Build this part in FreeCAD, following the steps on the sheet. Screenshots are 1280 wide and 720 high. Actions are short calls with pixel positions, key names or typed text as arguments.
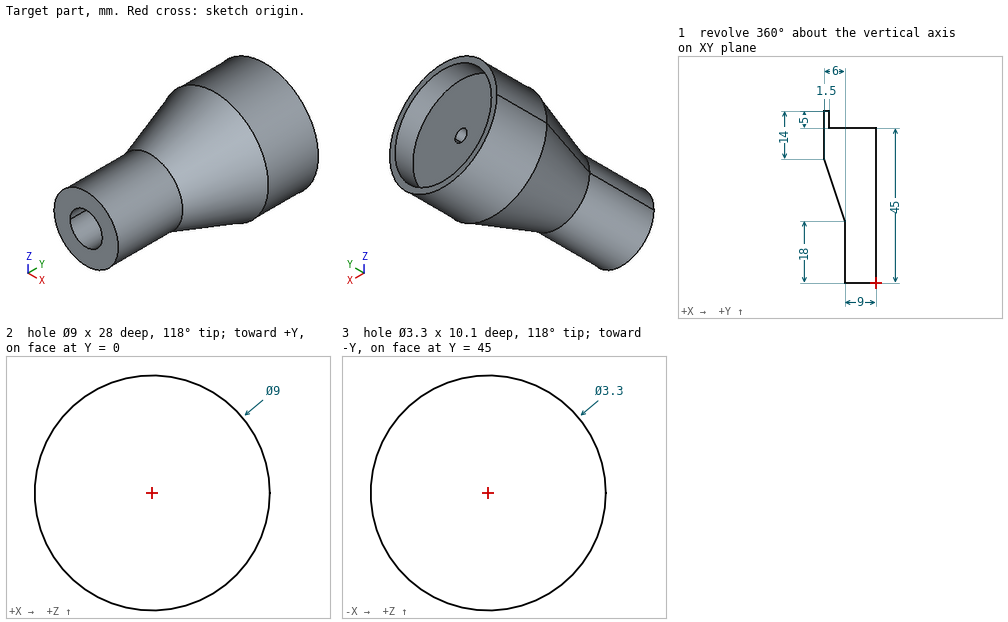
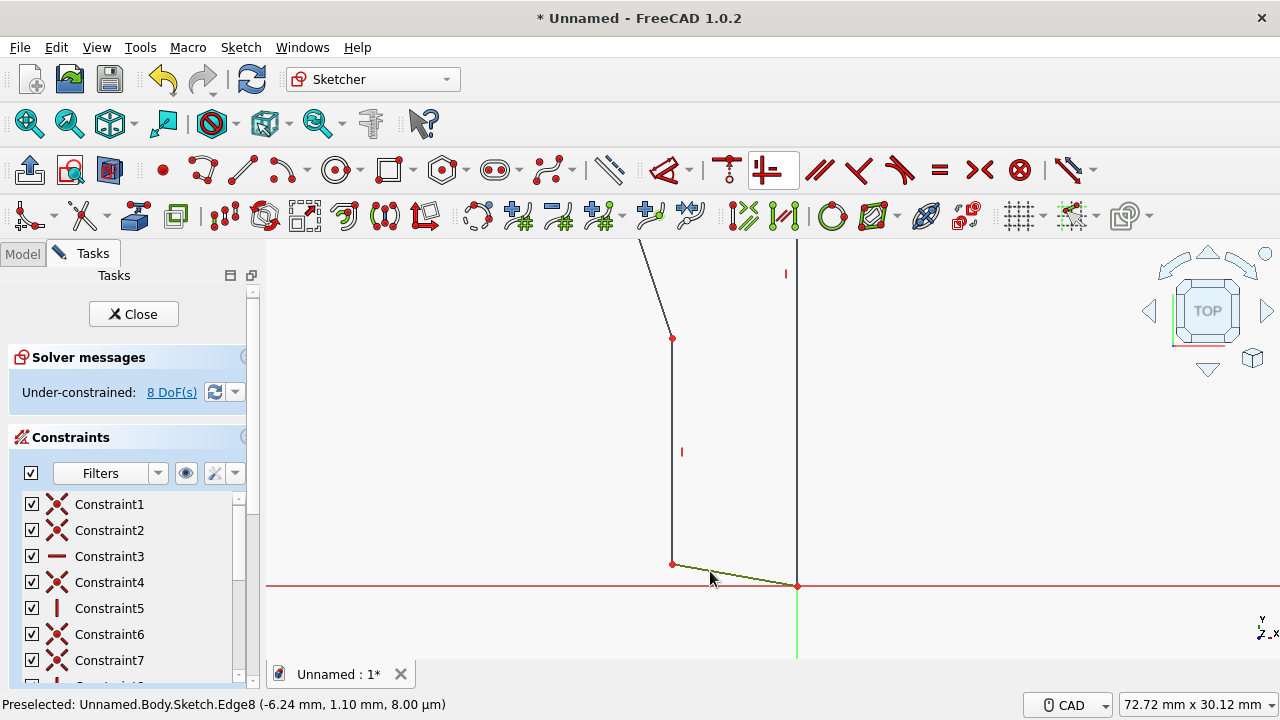
key(h)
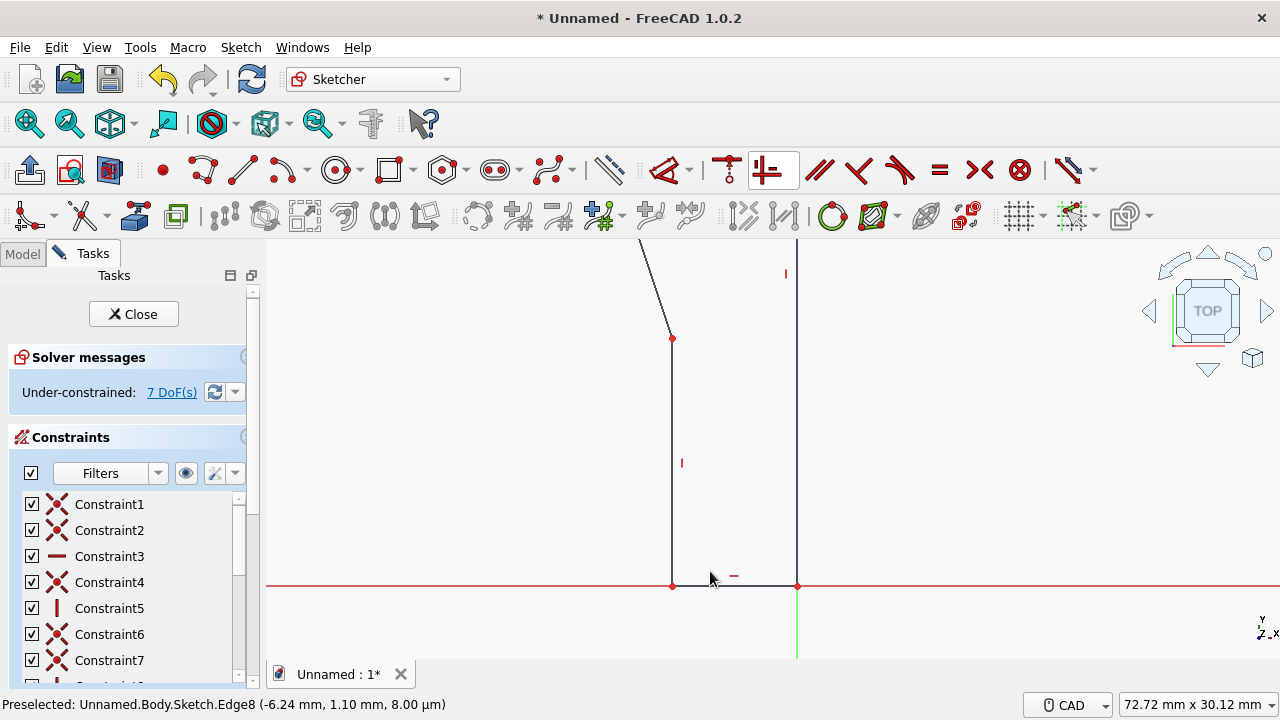
click(664, 170)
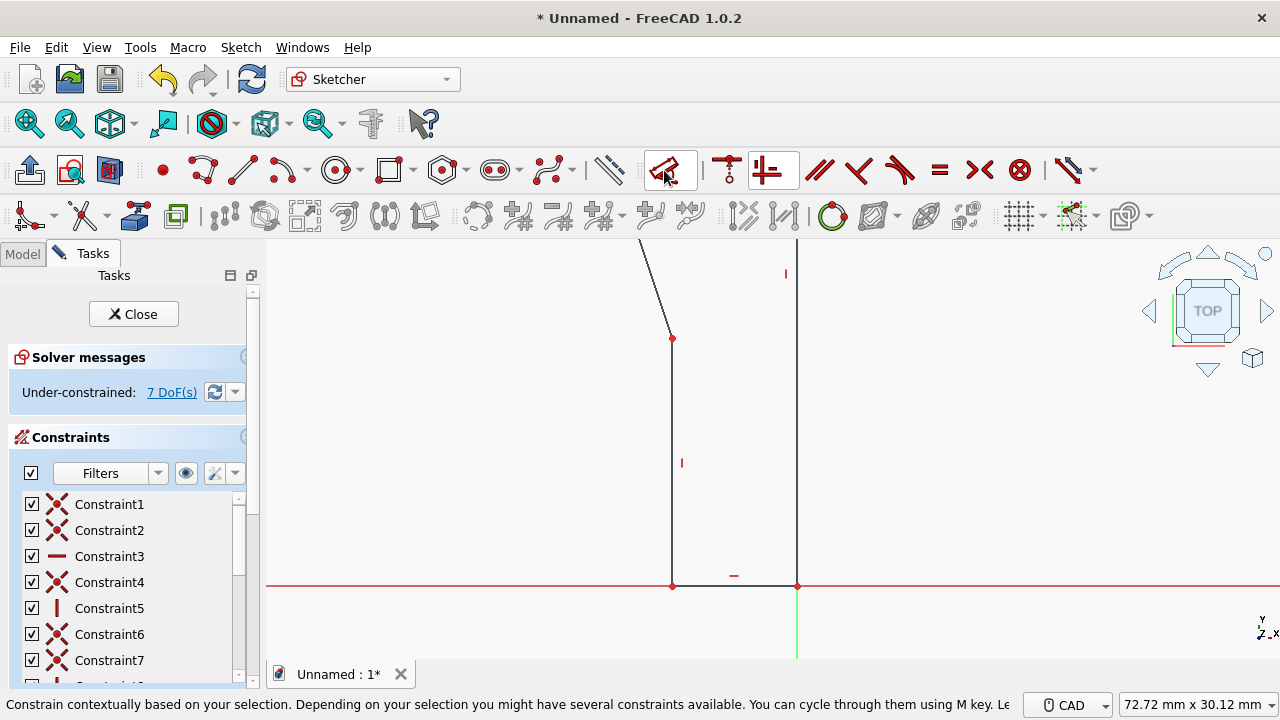
scroll(711, 572, down, 5)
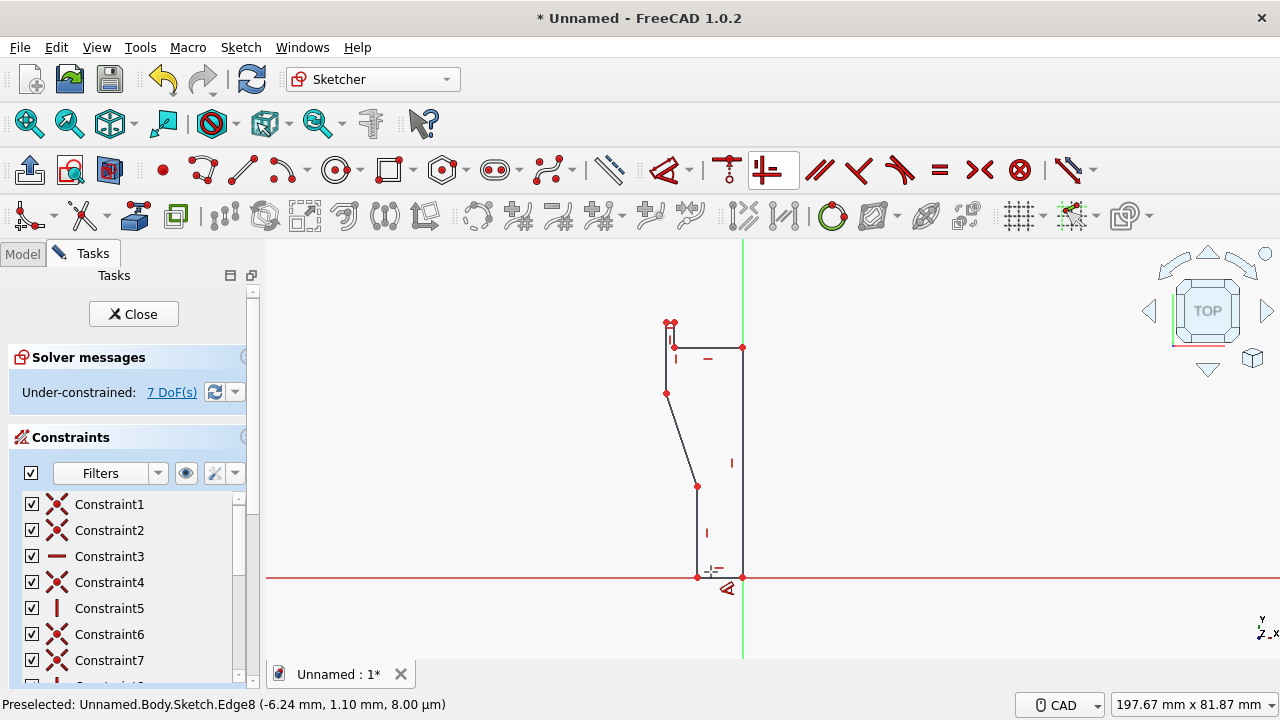
scroll(674, 340, up, 4)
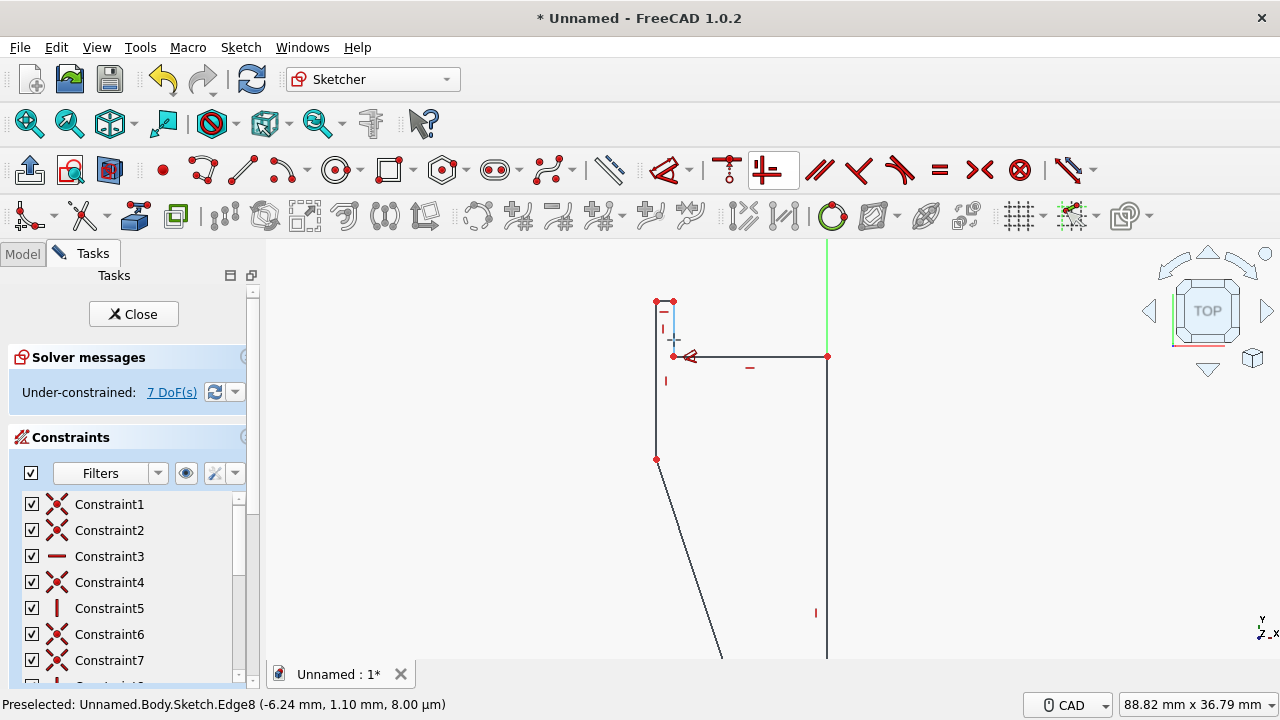
click(674, 340)
click(640, 329)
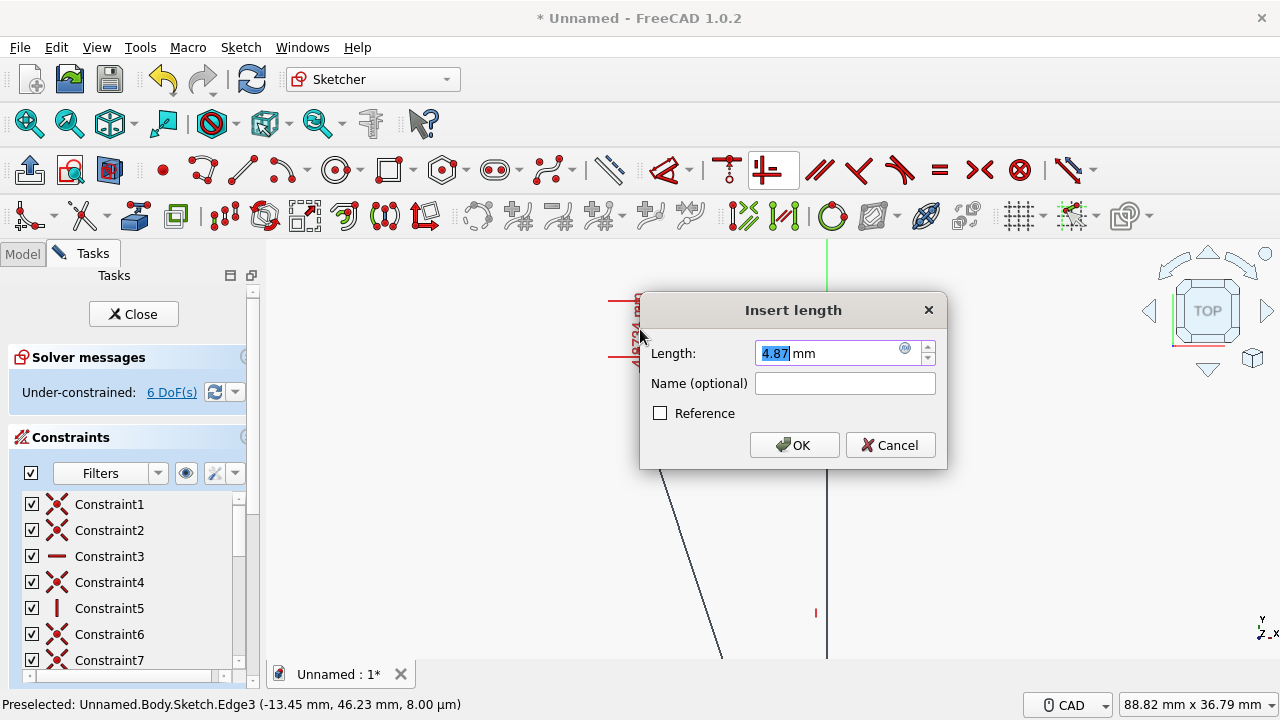
text(5)
key(Return)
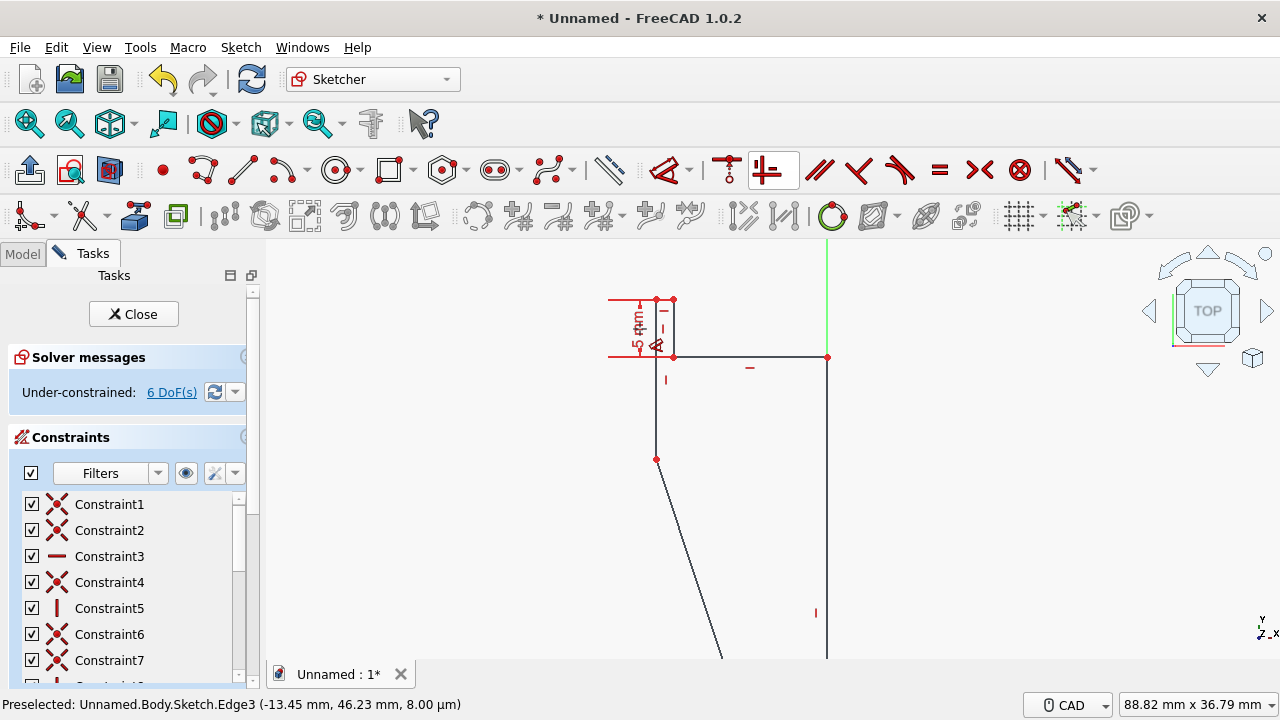
scroll(674, 339, down, 4)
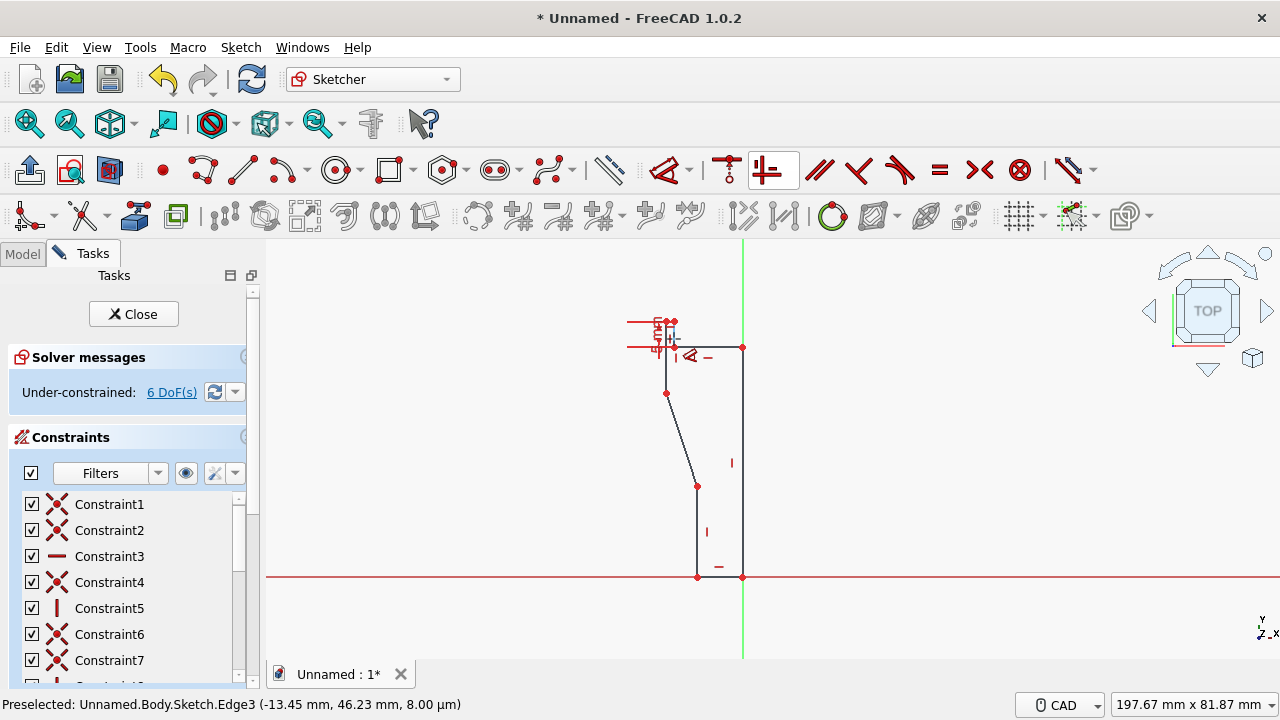
click(711, 577)
click(720, 611)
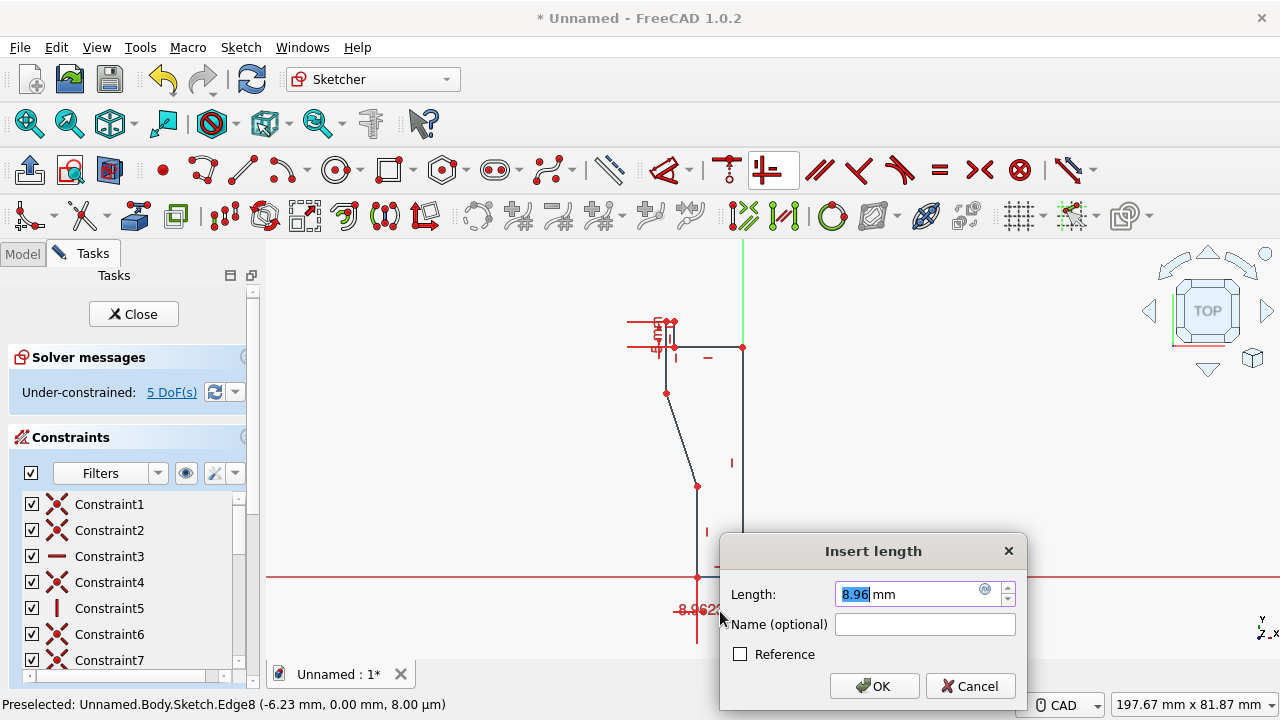
text(9)
key(Return)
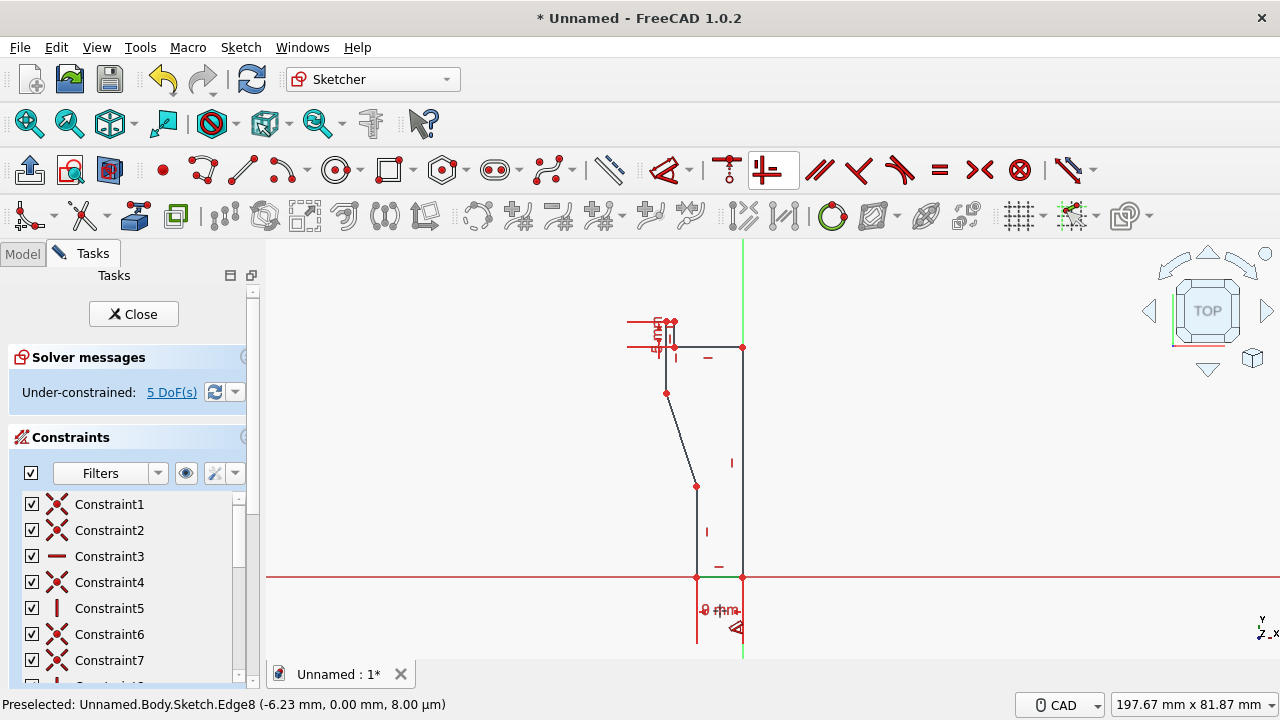
click(743, 508)
click(777, 462)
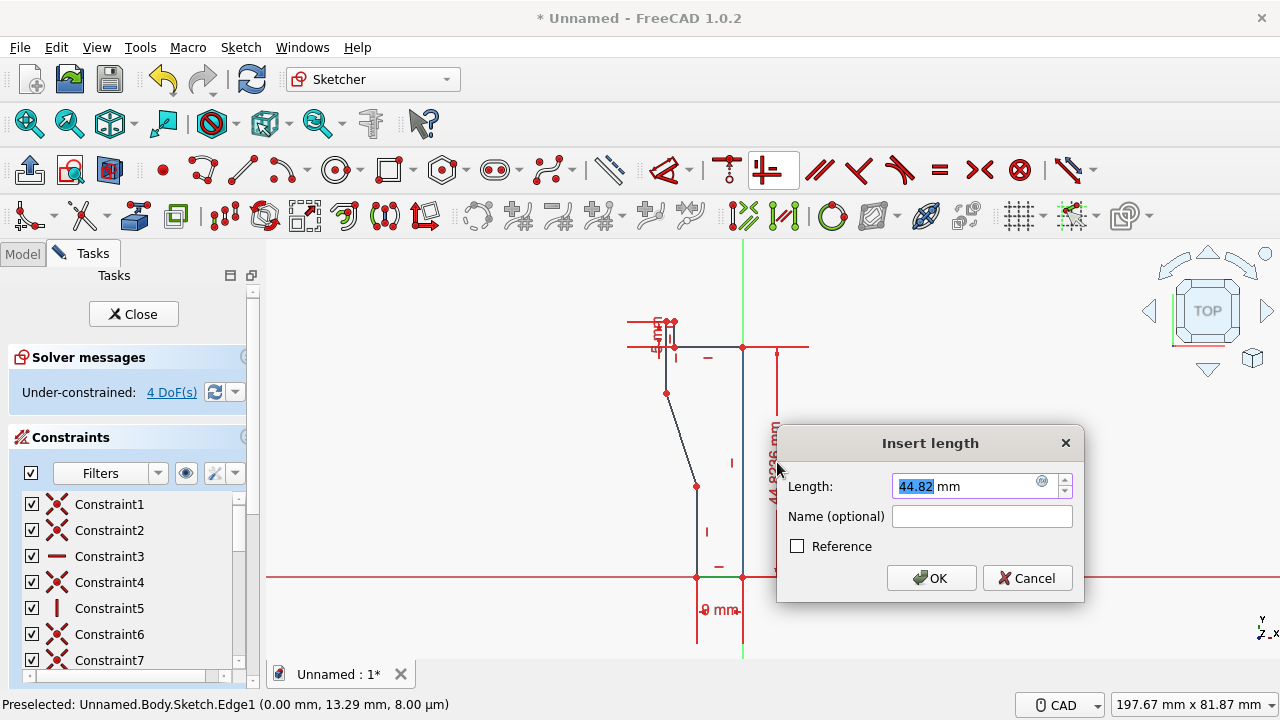
text(45)
key(Return)